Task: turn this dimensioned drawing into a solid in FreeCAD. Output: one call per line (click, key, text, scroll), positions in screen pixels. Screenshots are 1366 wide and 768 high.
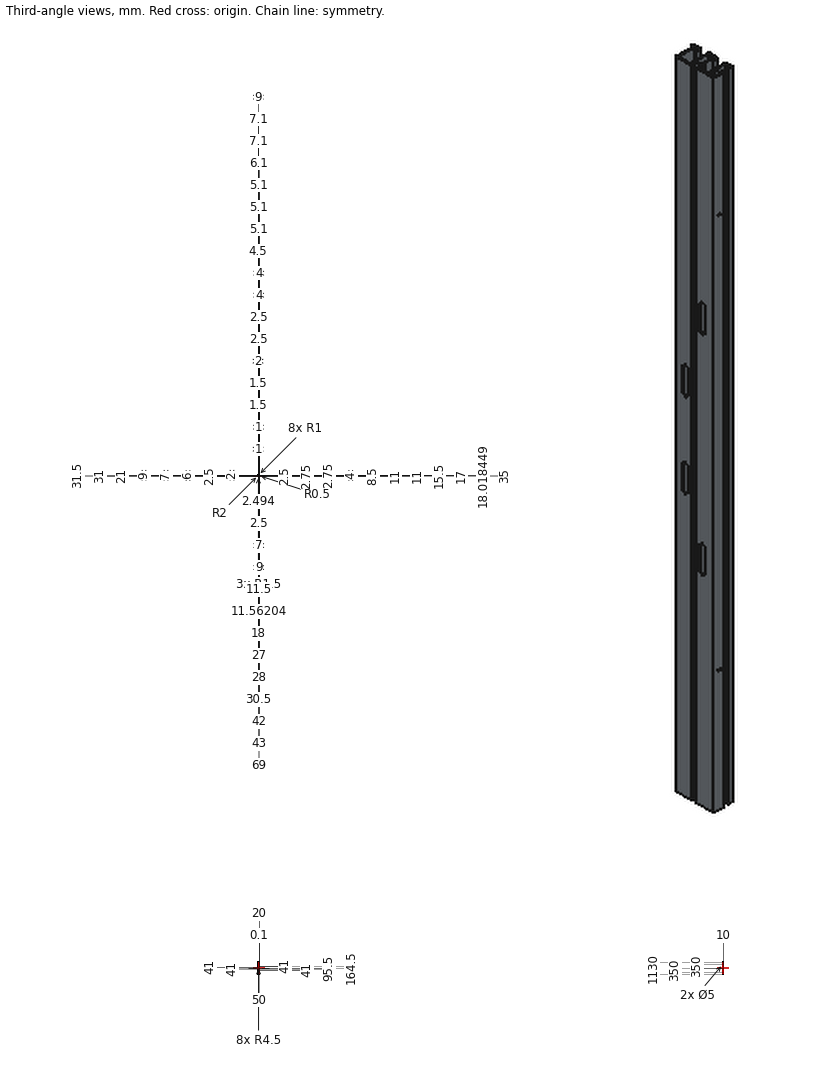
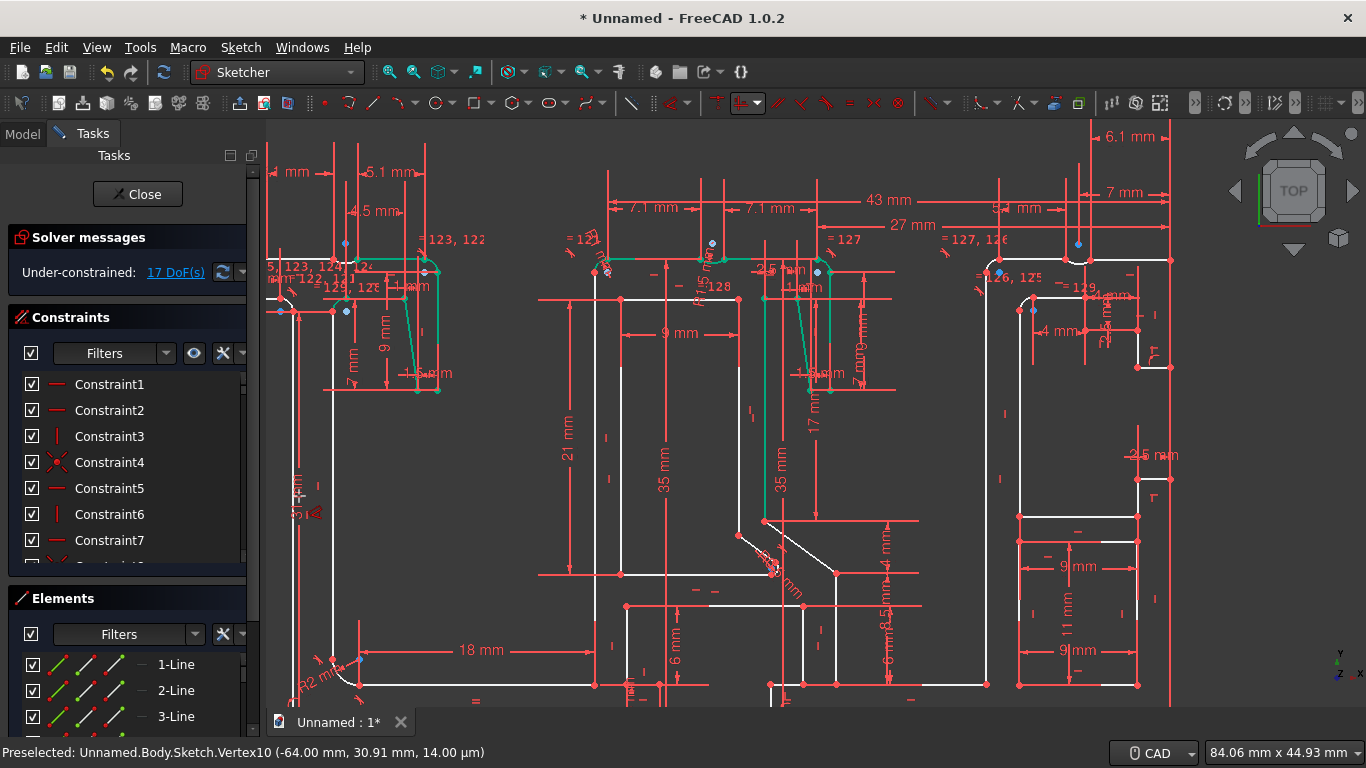
scroll(819, 260, down, 2)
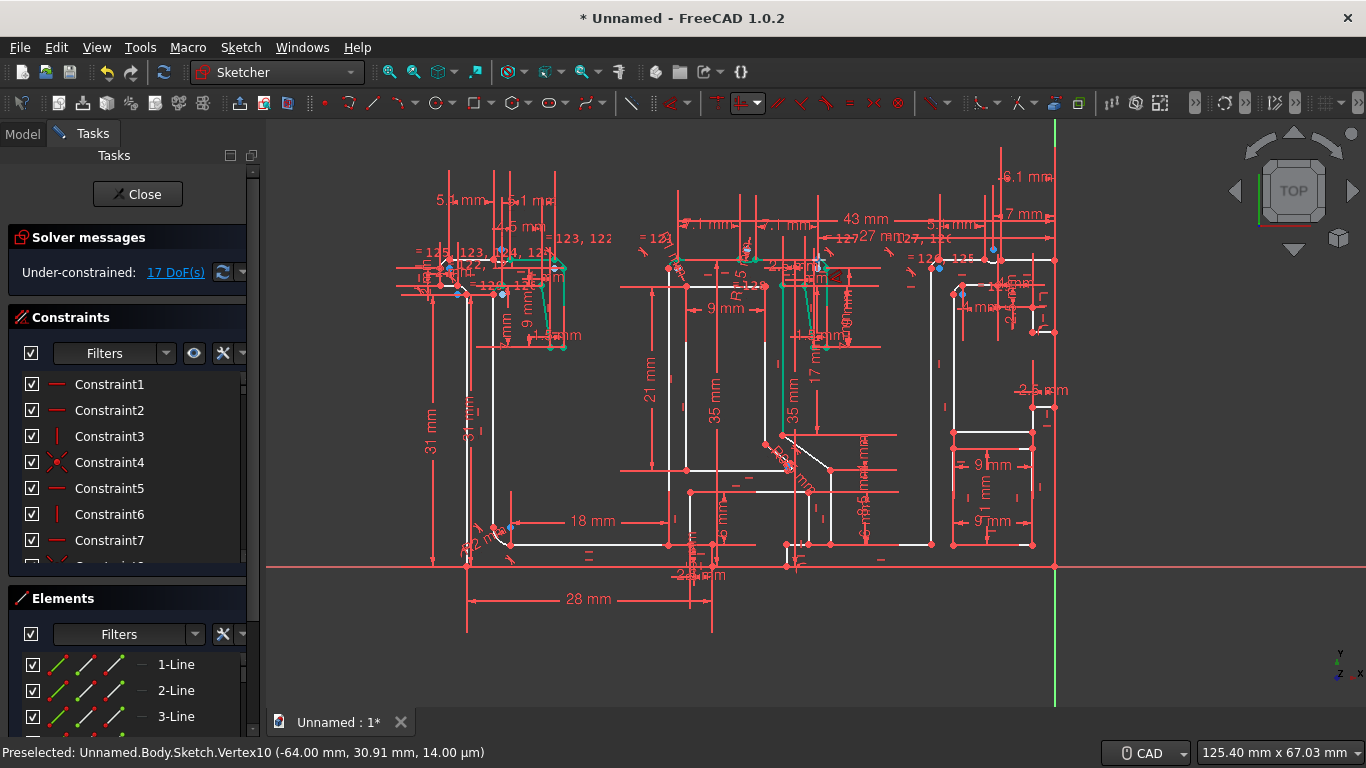
scroll(449, 260, up, 2)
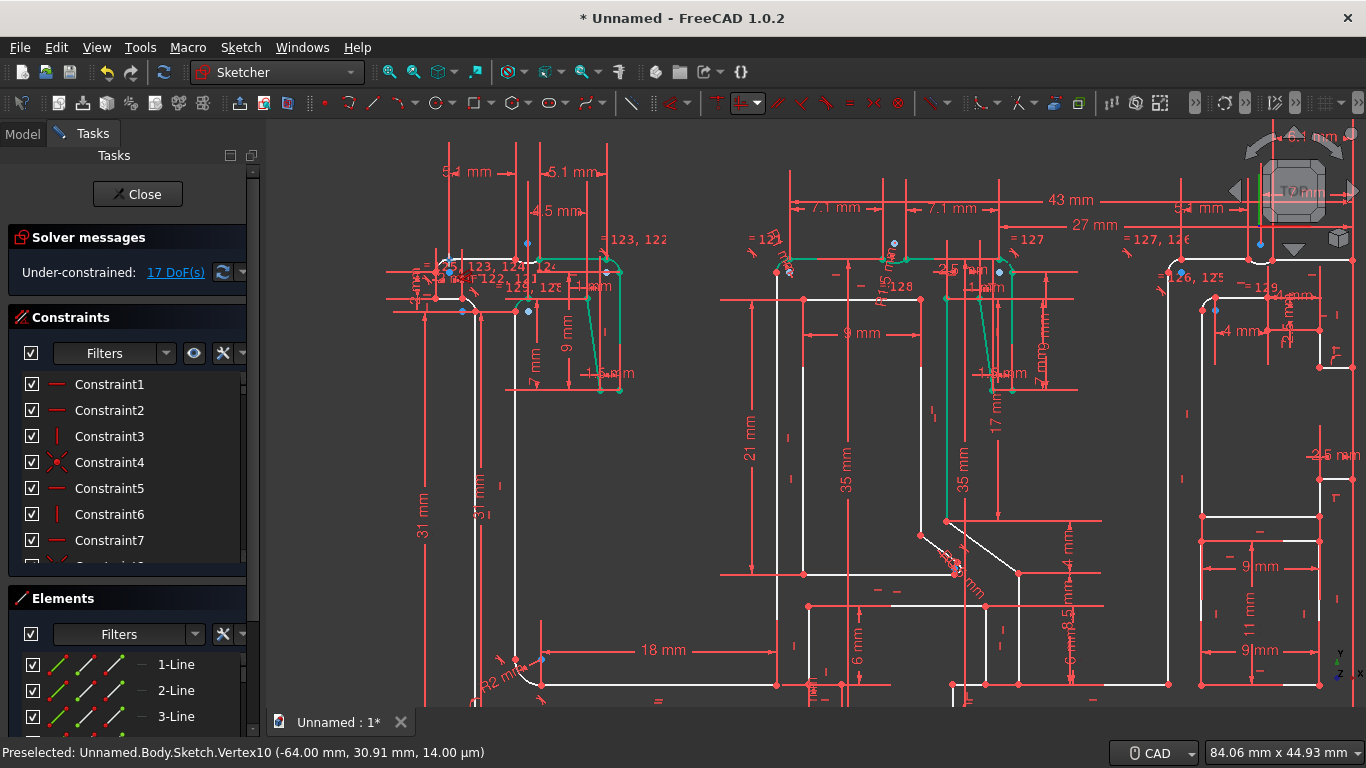
click(449, 259)
click(652, 225)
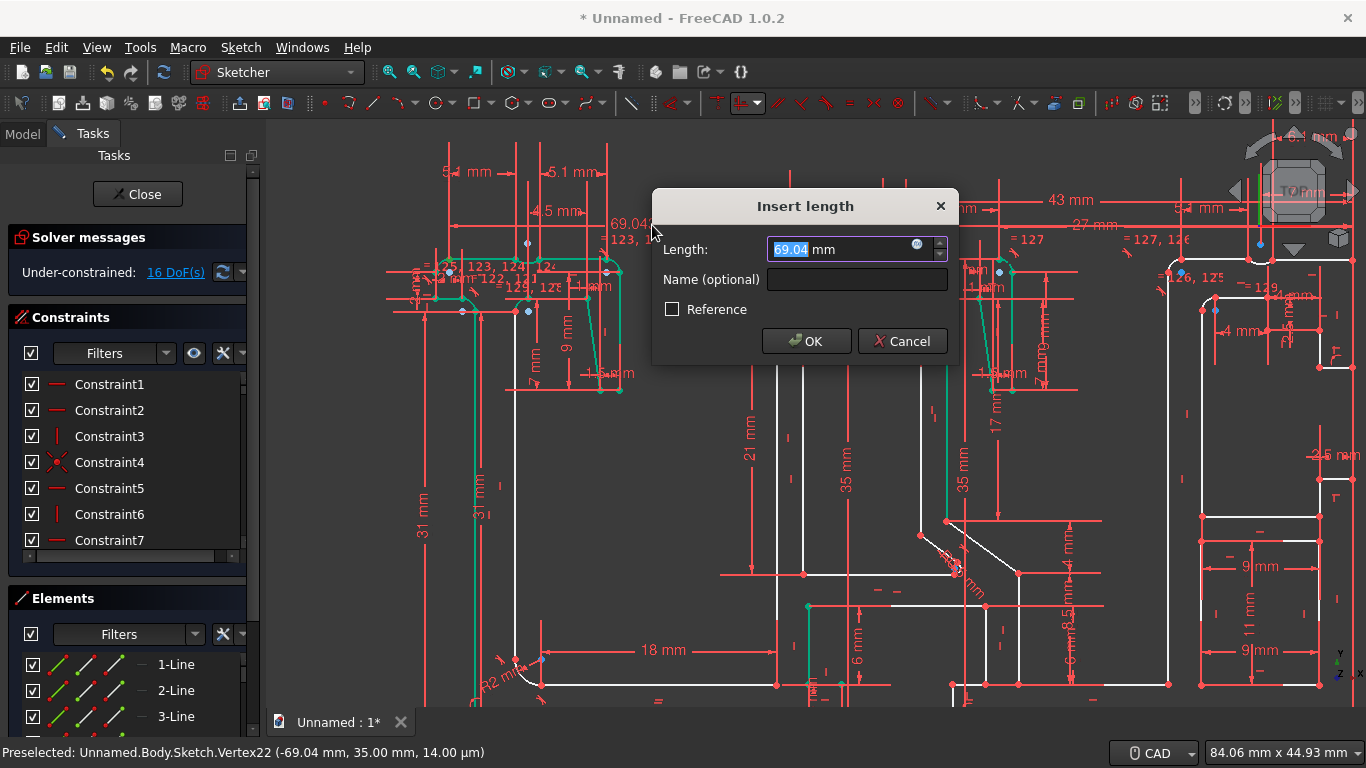
text(69)
key(Return)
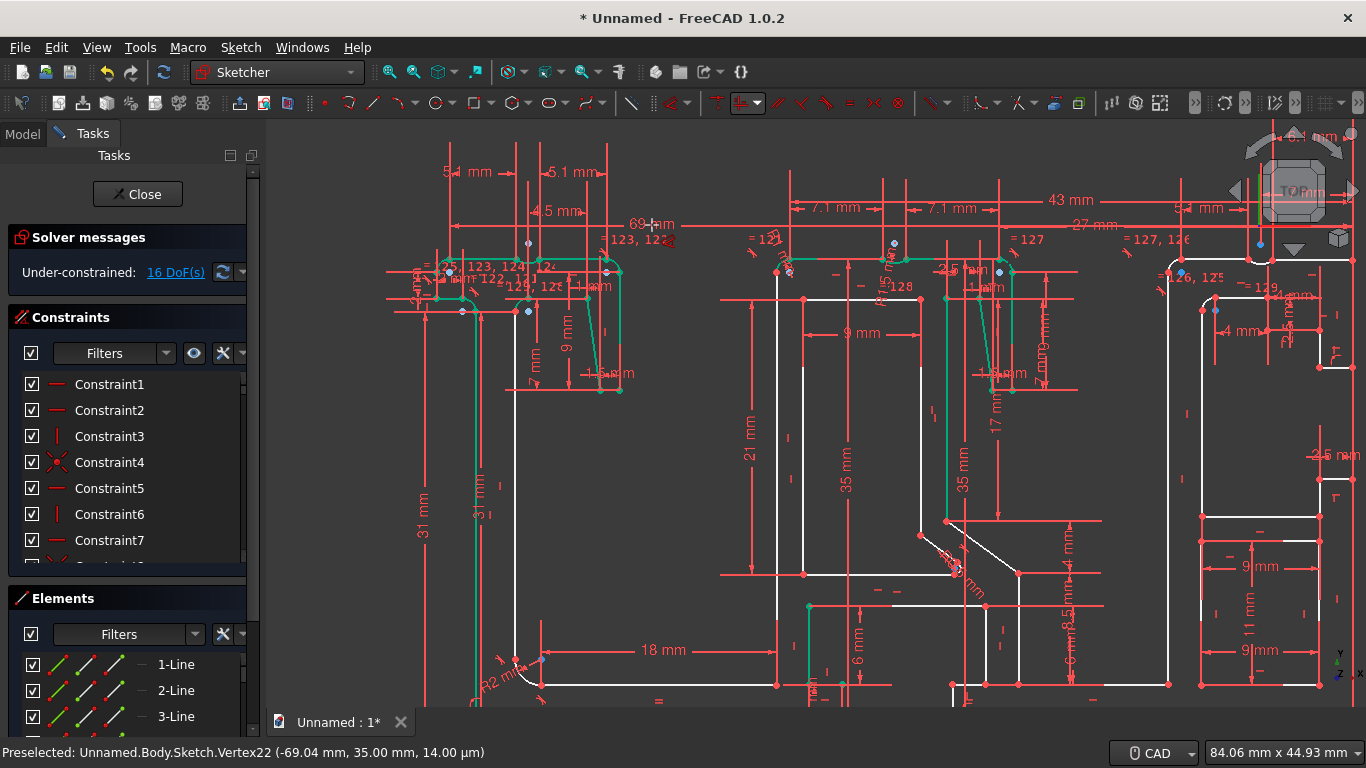
scroll(448, 260, down, 2)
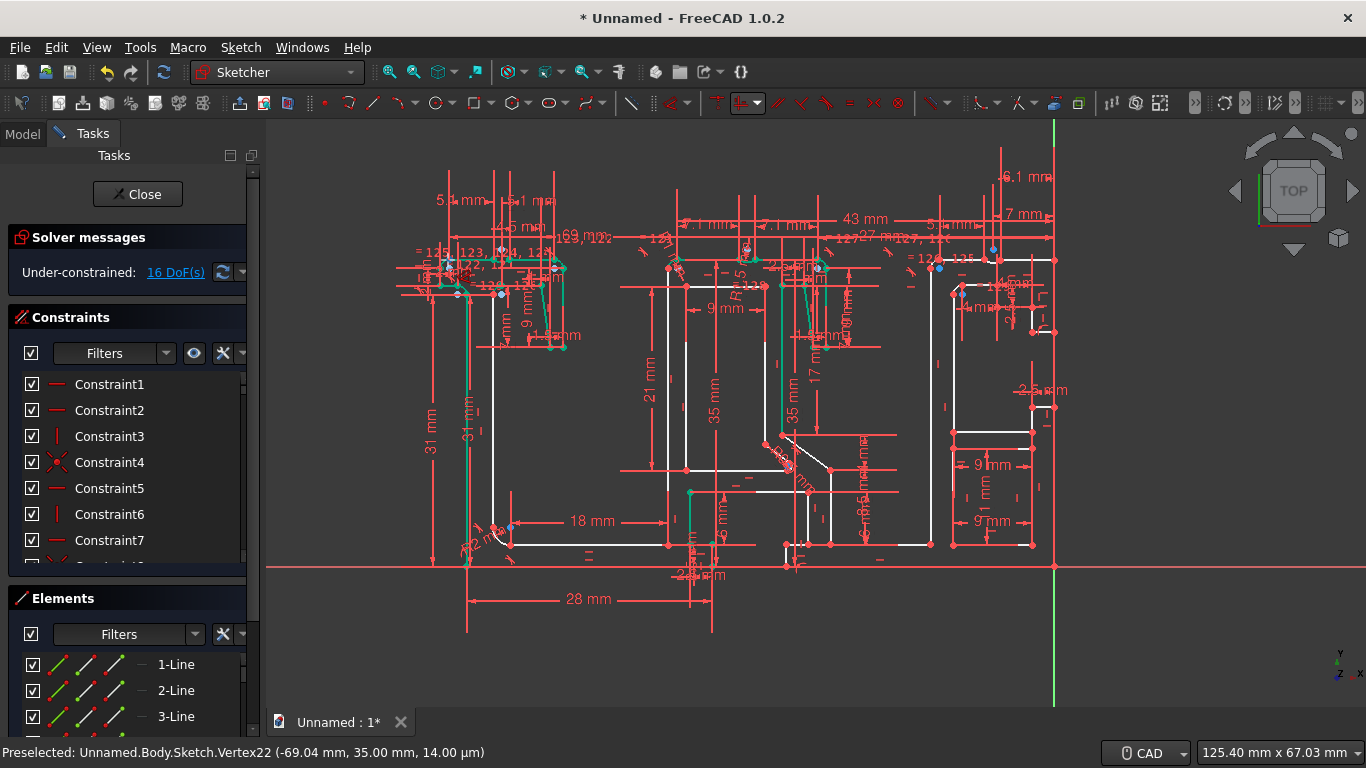
scroll(954, 294, up, 2)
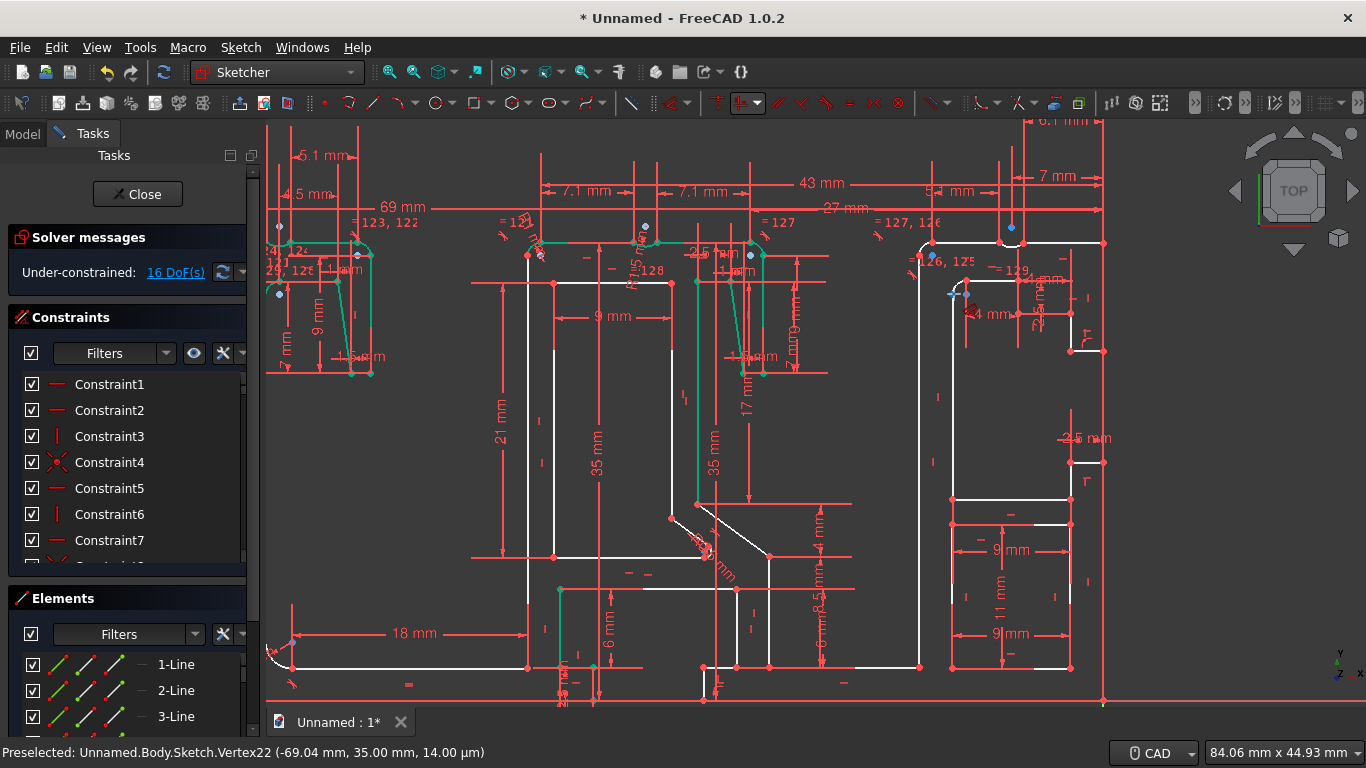
click(953, 294)
click(1137, 487)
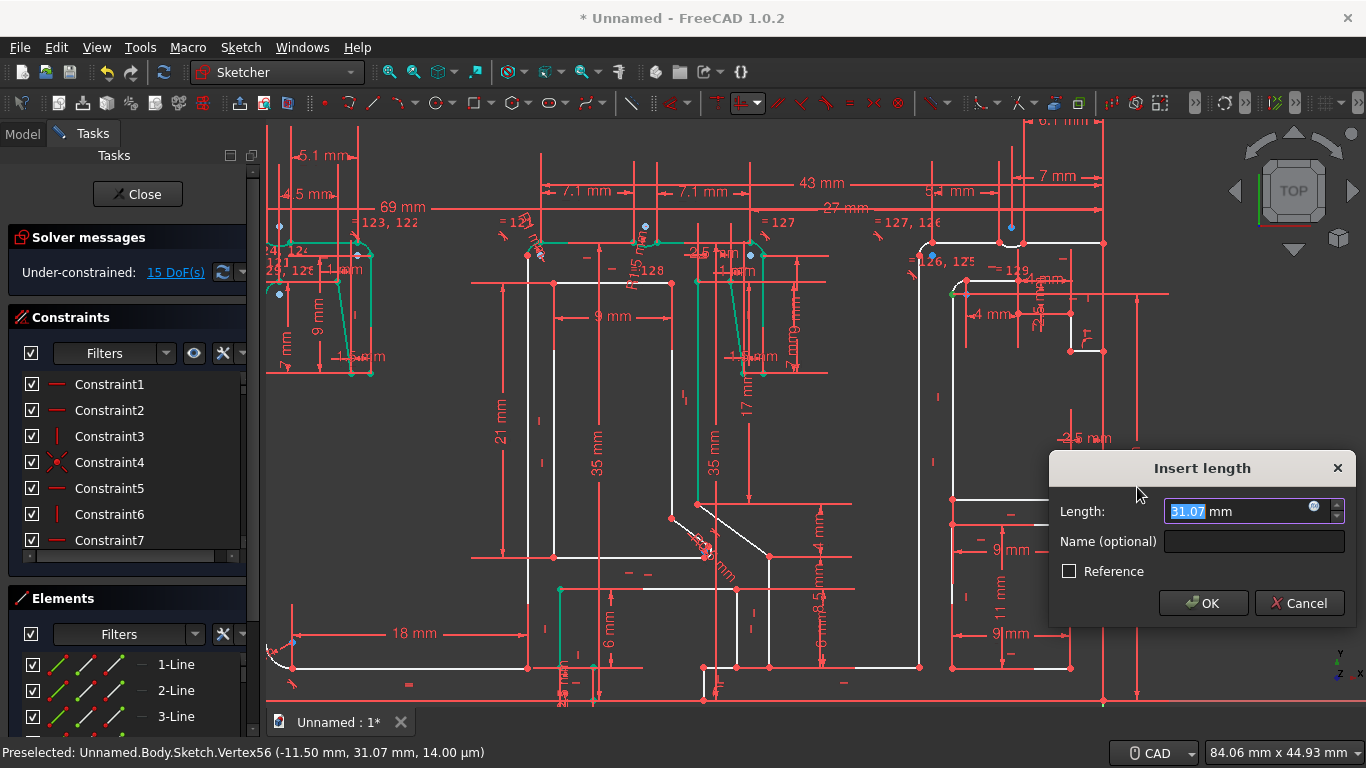
text(31)
key(Return)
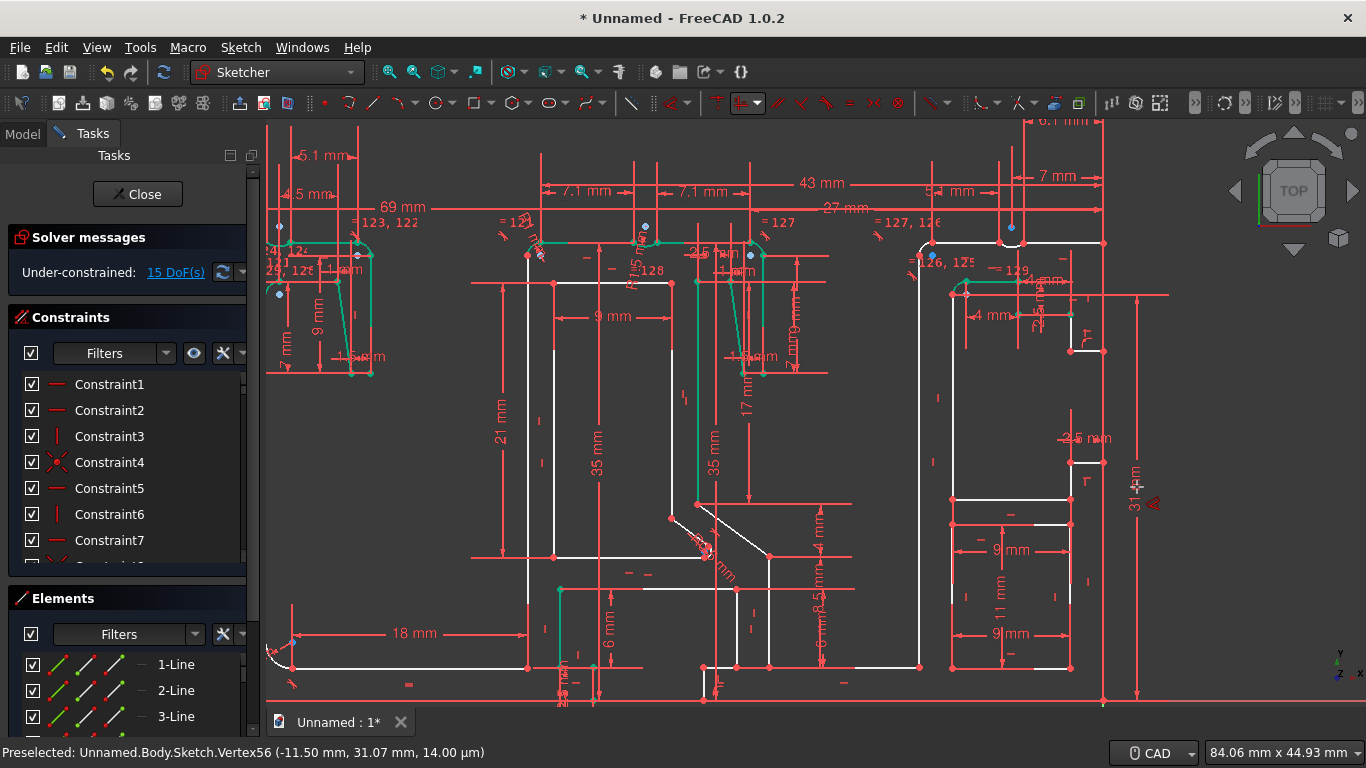
click(1103, 243)
click(1137, 461)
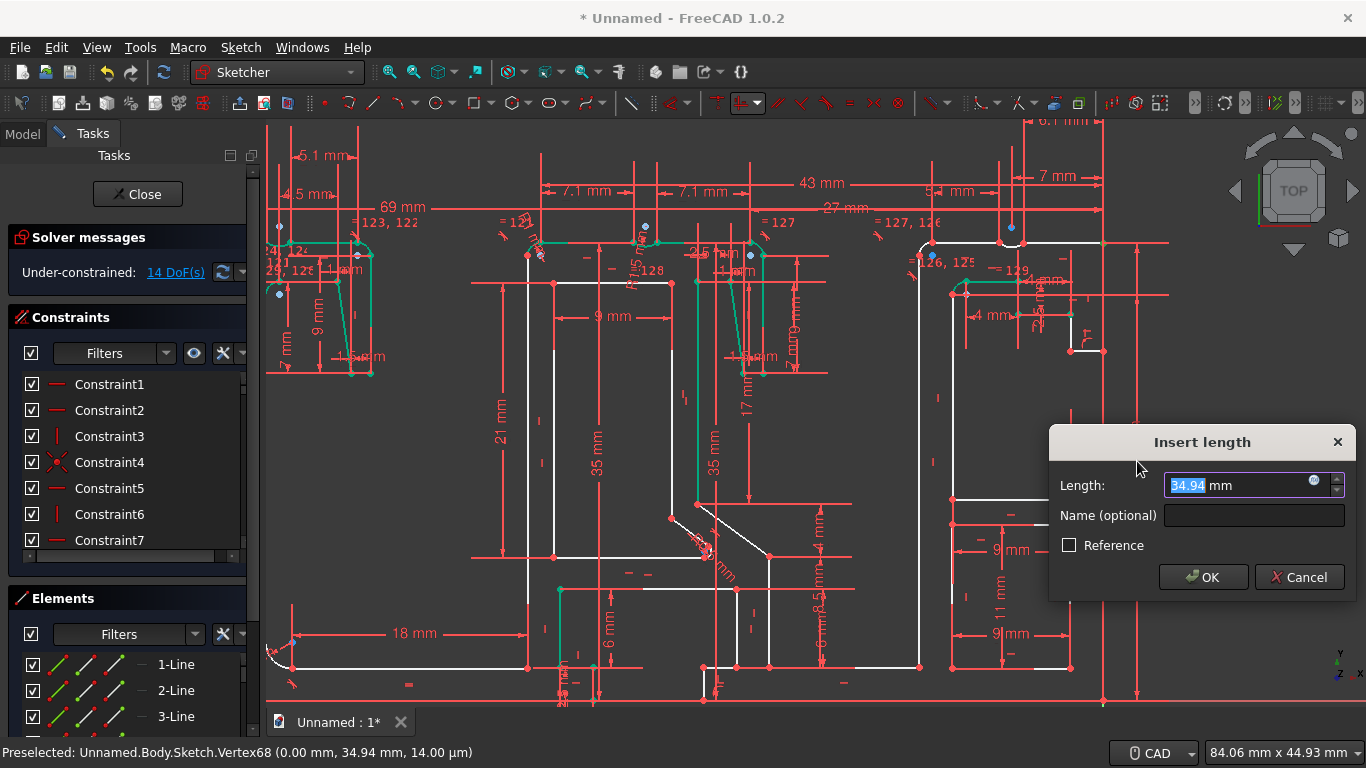
text(35)
key(Return)